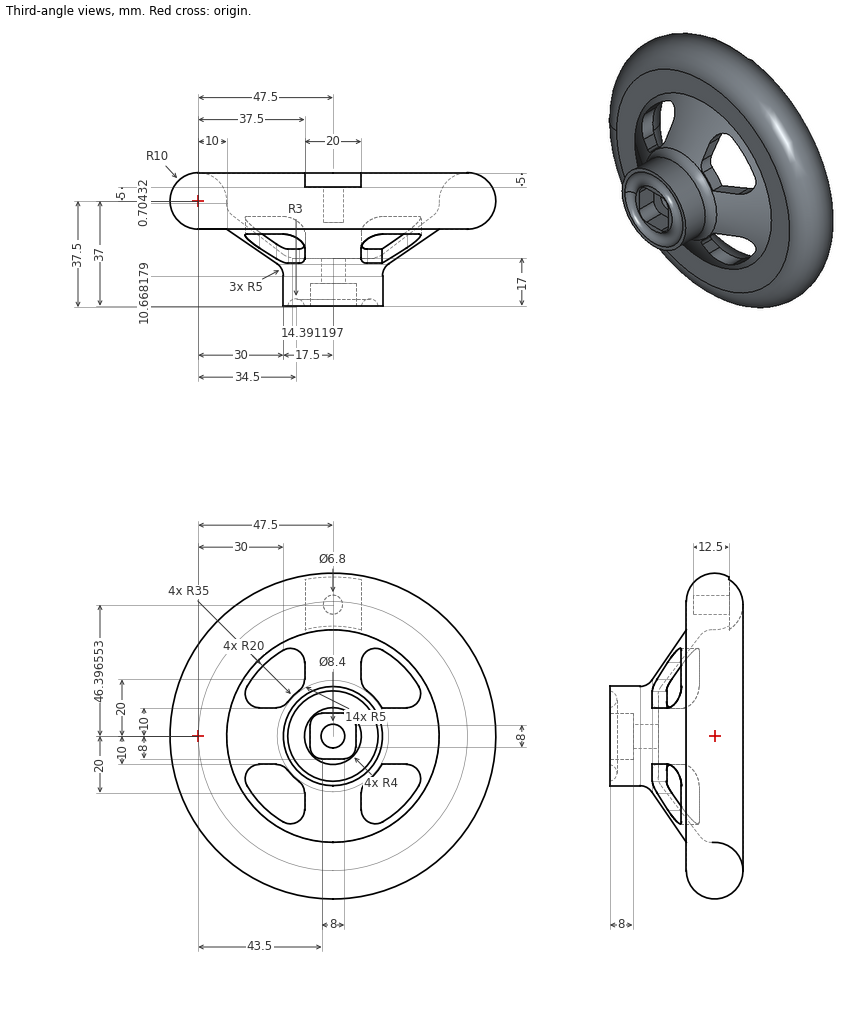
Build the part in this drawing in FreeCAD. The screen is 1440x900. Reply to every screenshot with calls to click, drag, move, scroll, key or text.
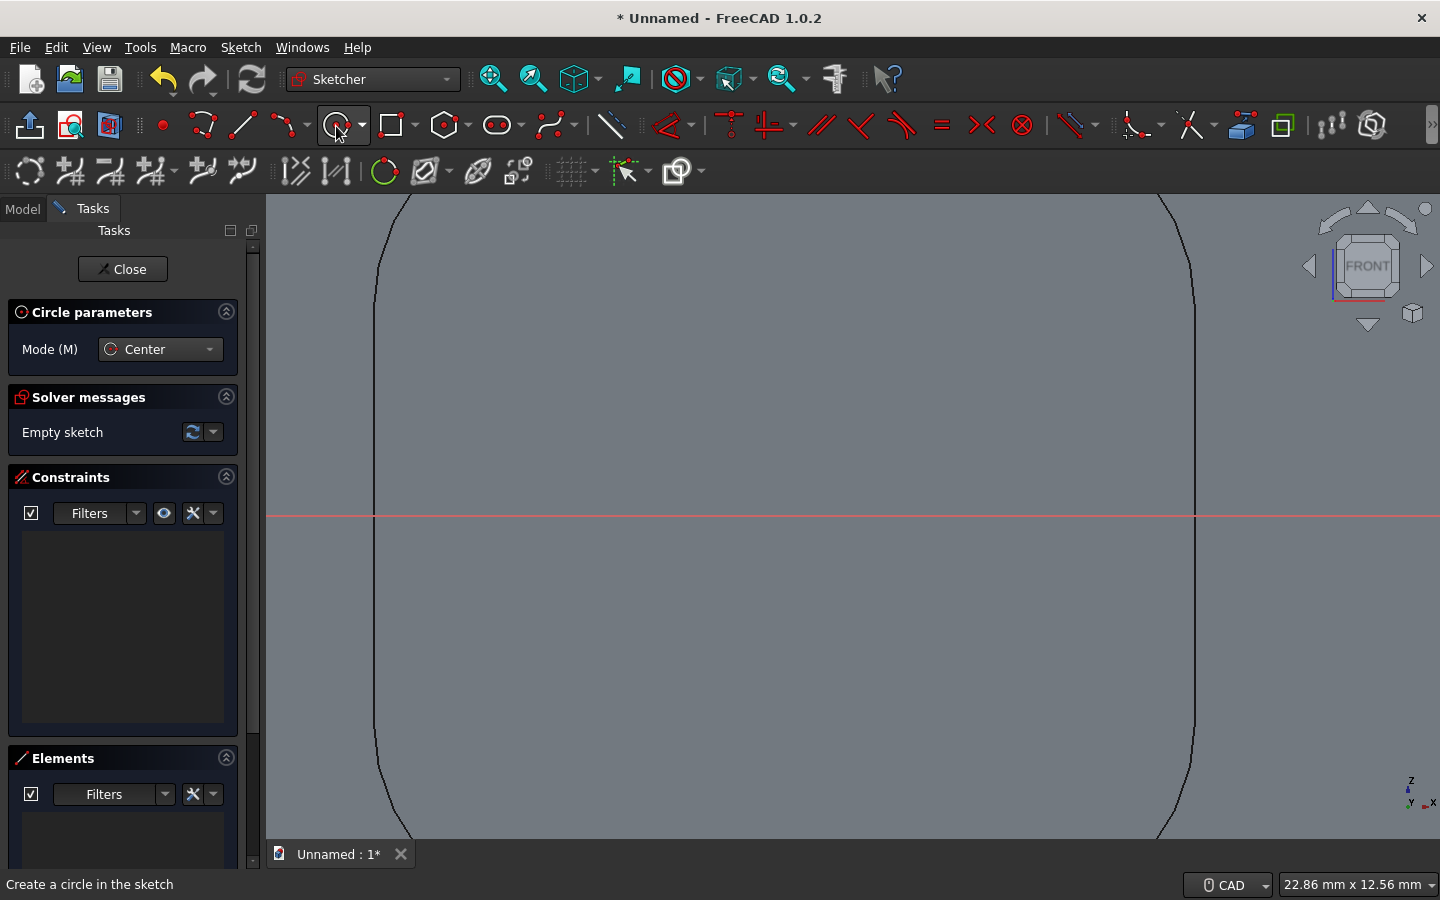
click(784, 516)
move(937, 363)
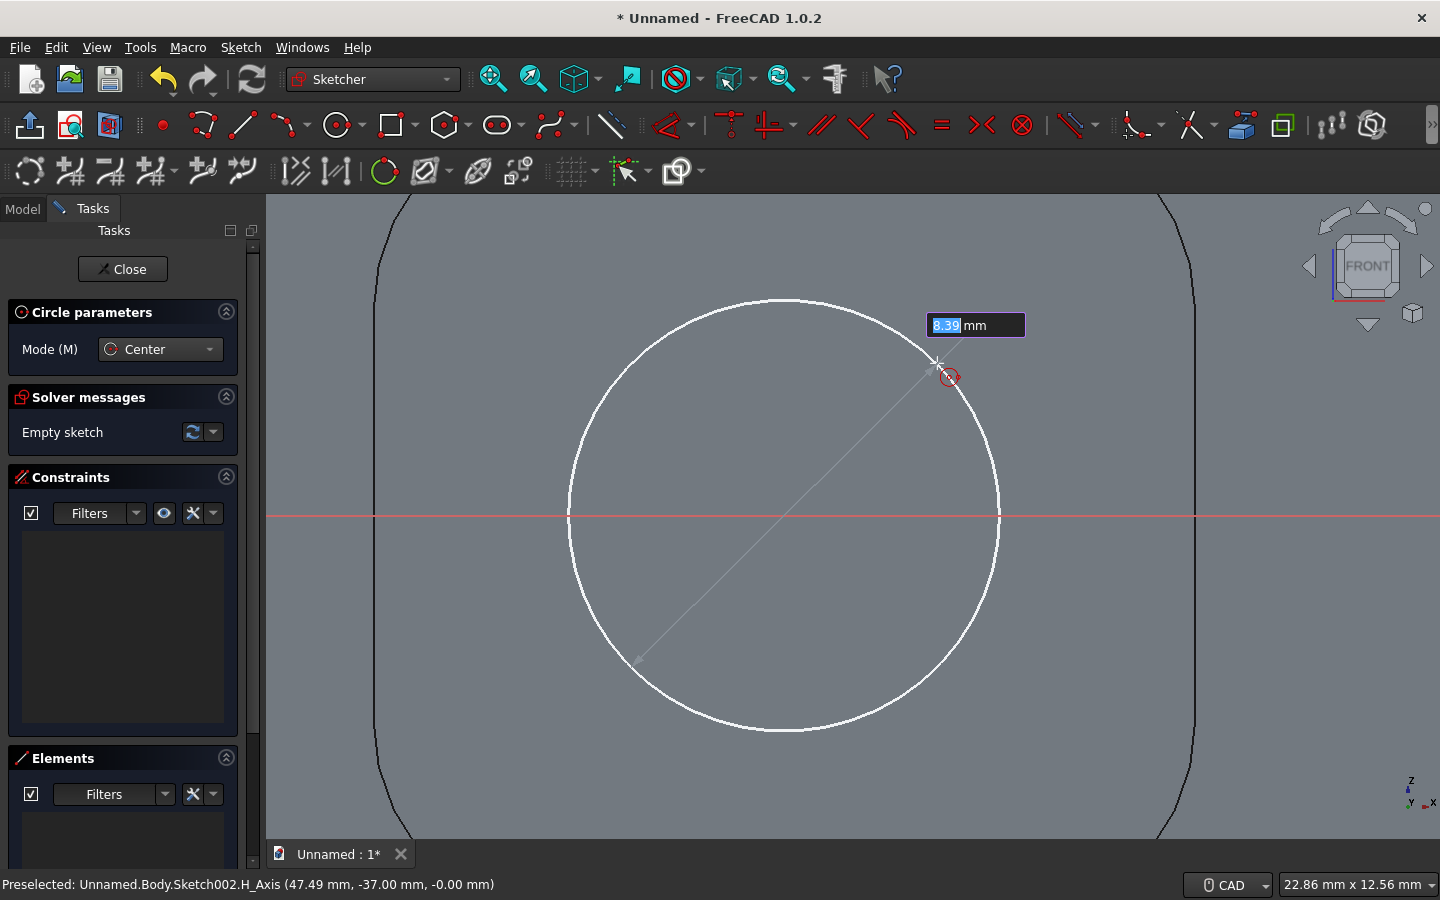
text(8.4)
key(Return)
key(Escape)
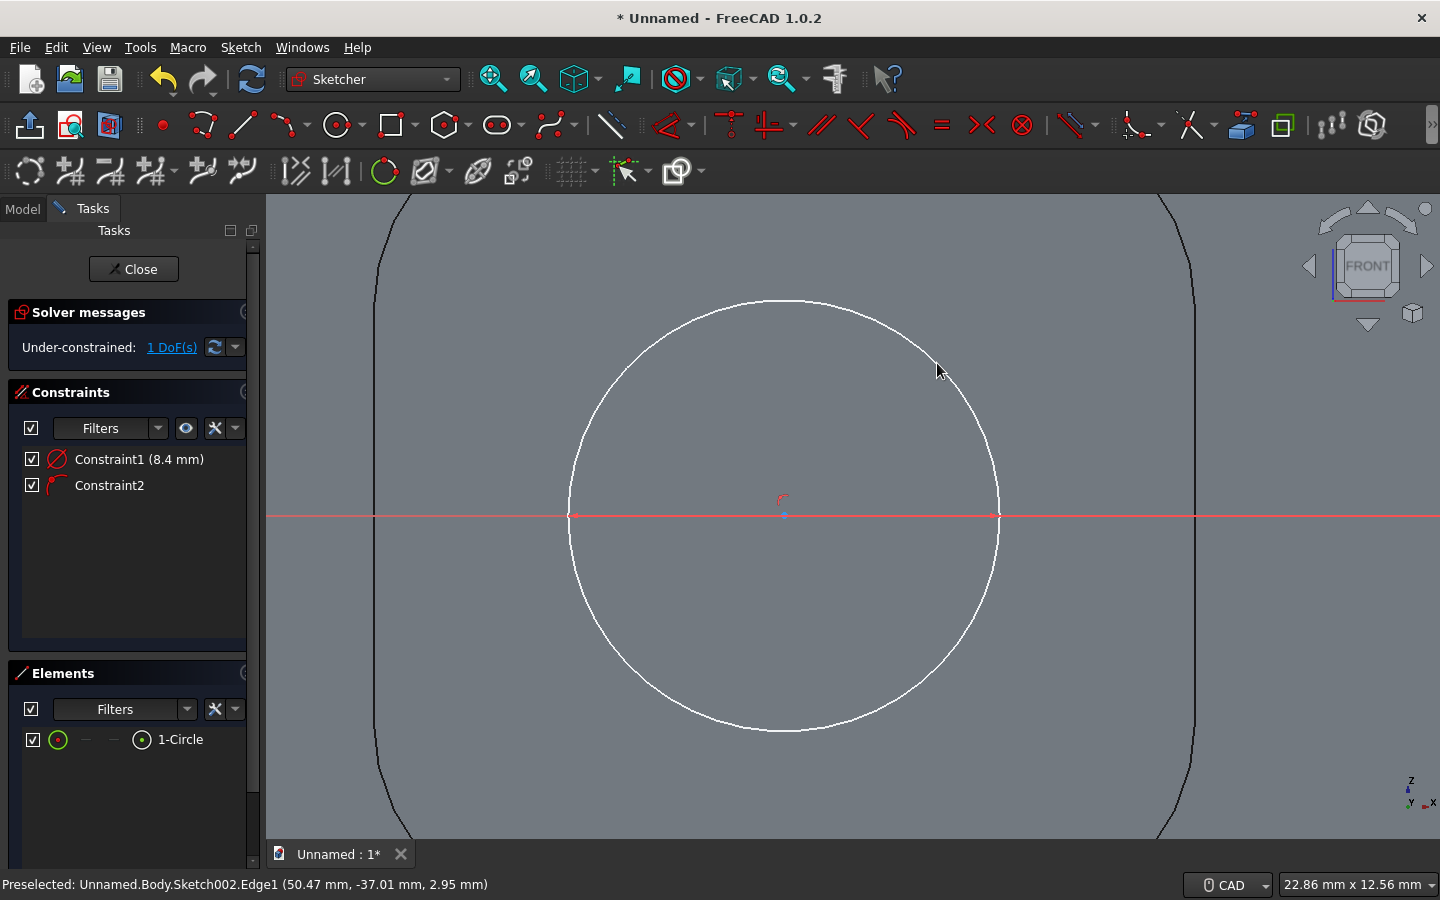
click(666, 126)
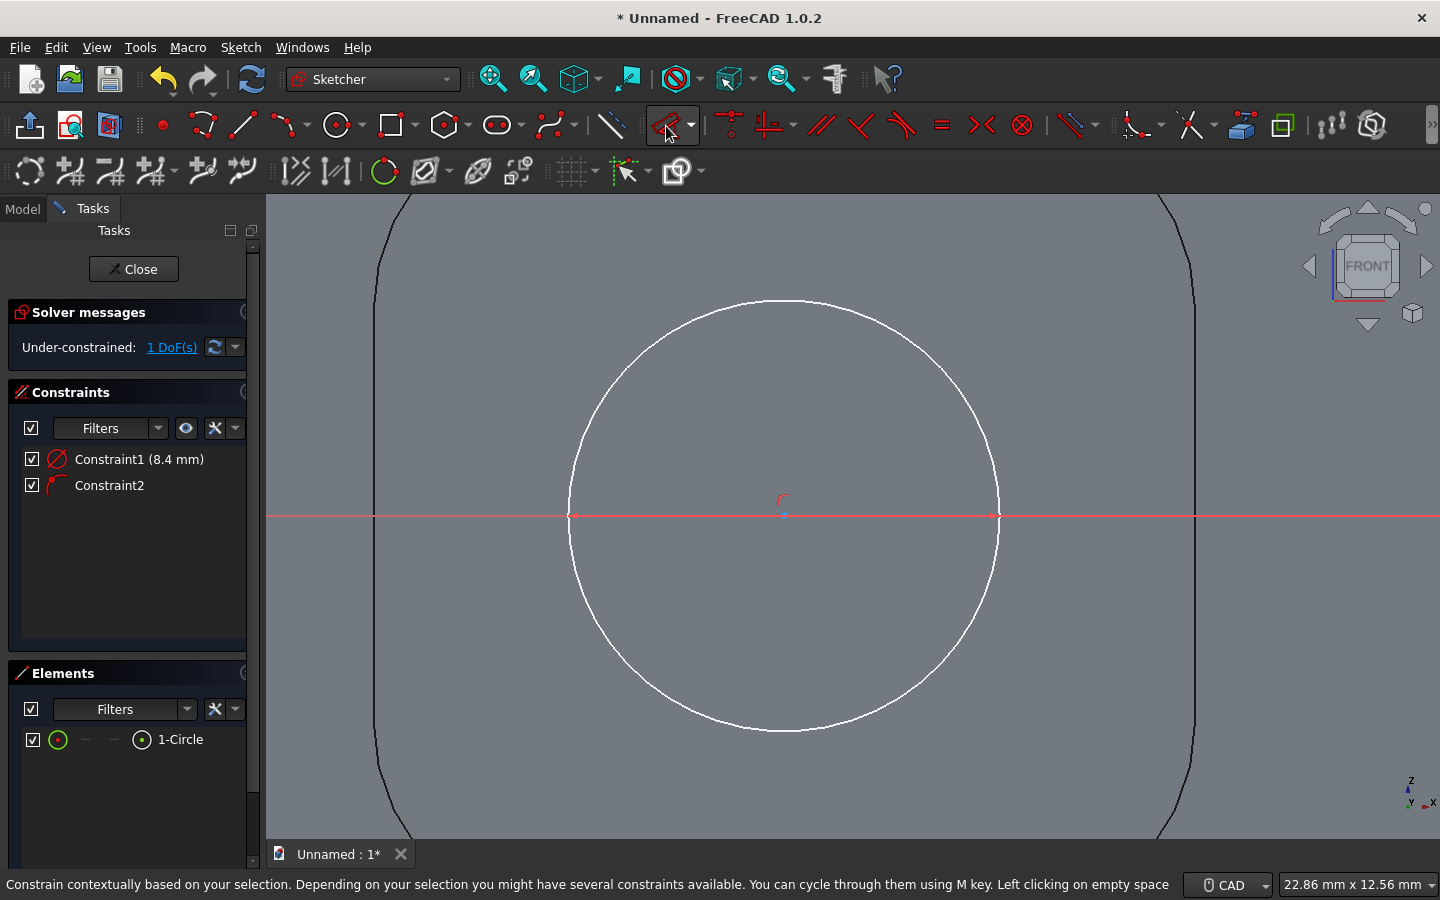
click(784, 516)
click(539, 550)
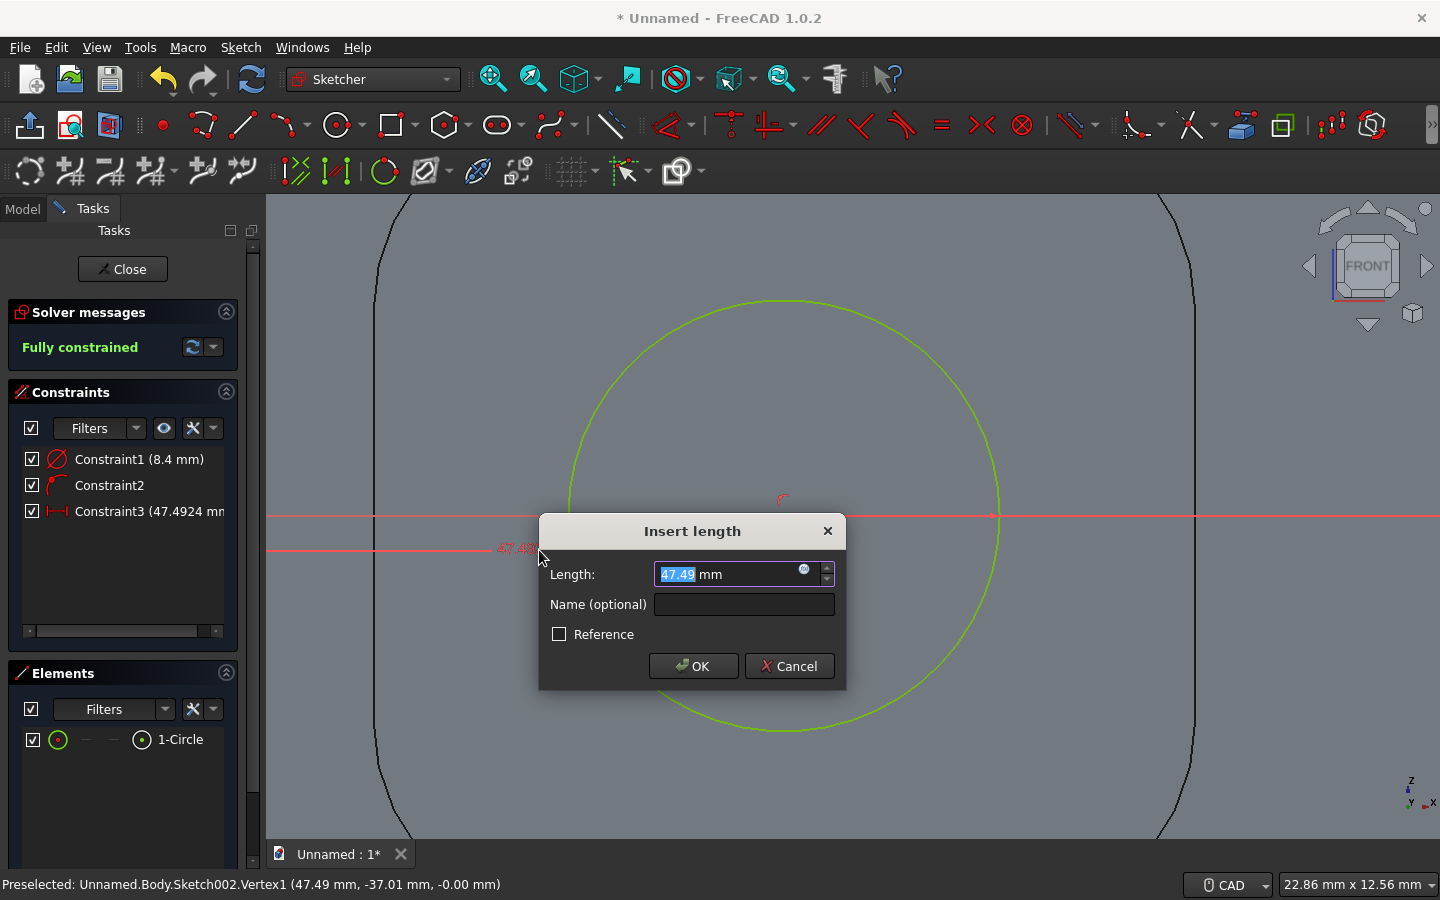
text(47.5)
key(Return)
key(Escape)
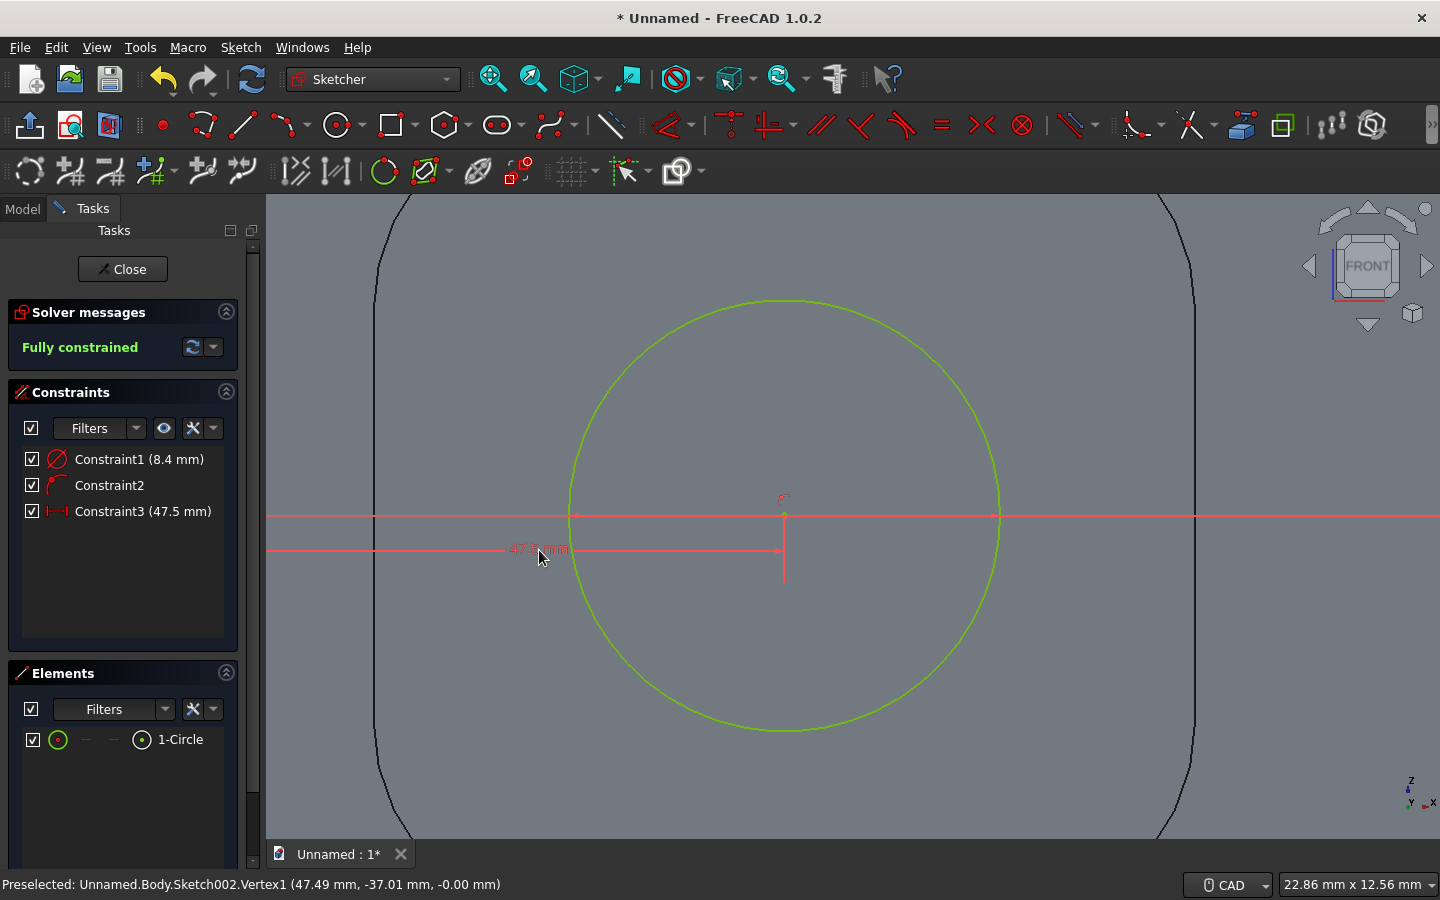
click(123, 269)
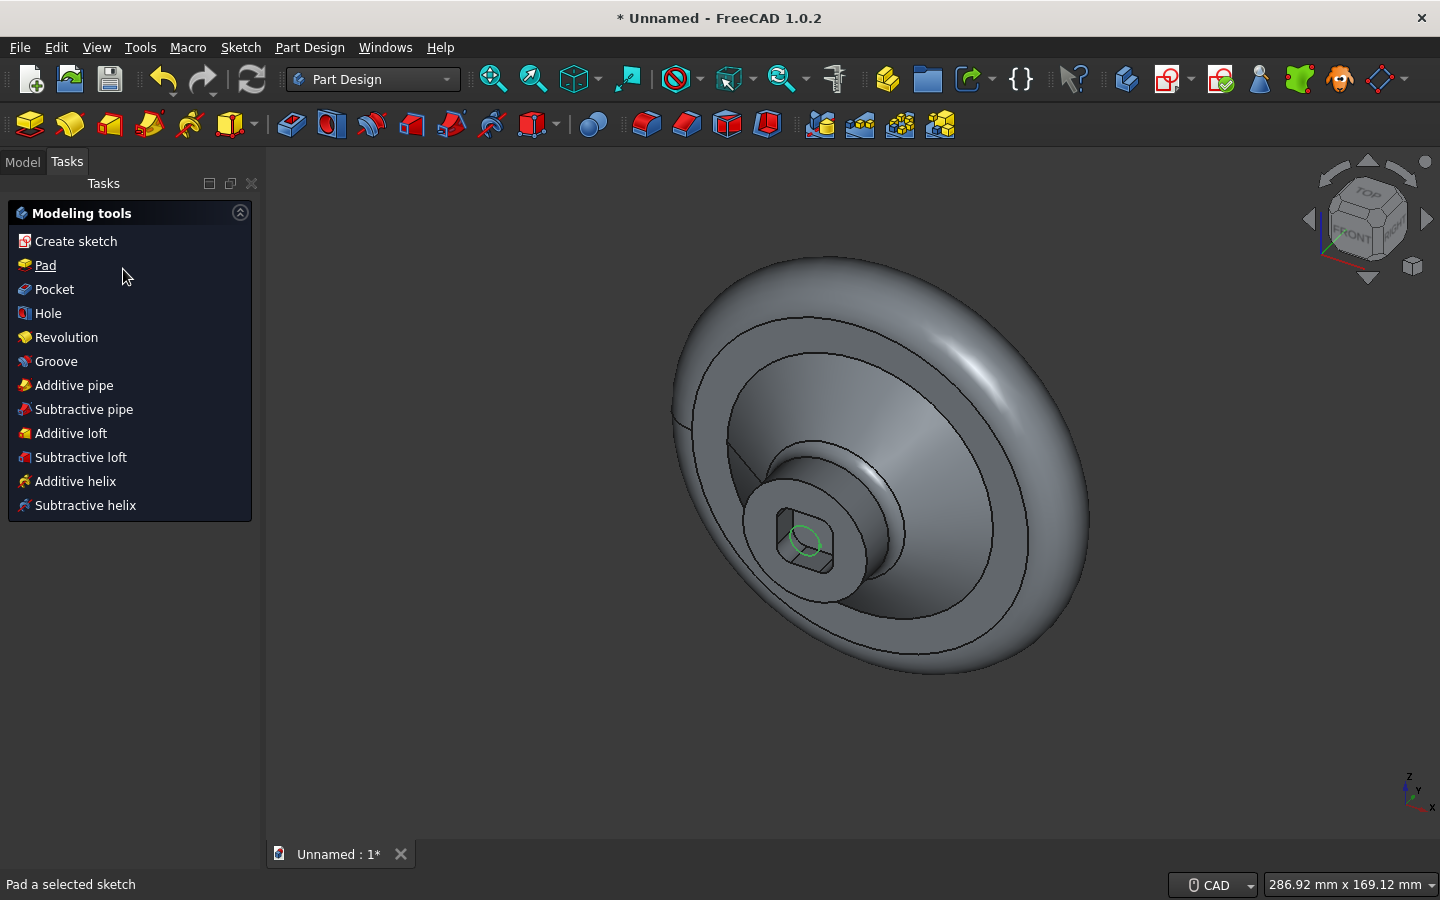
click(292, 124)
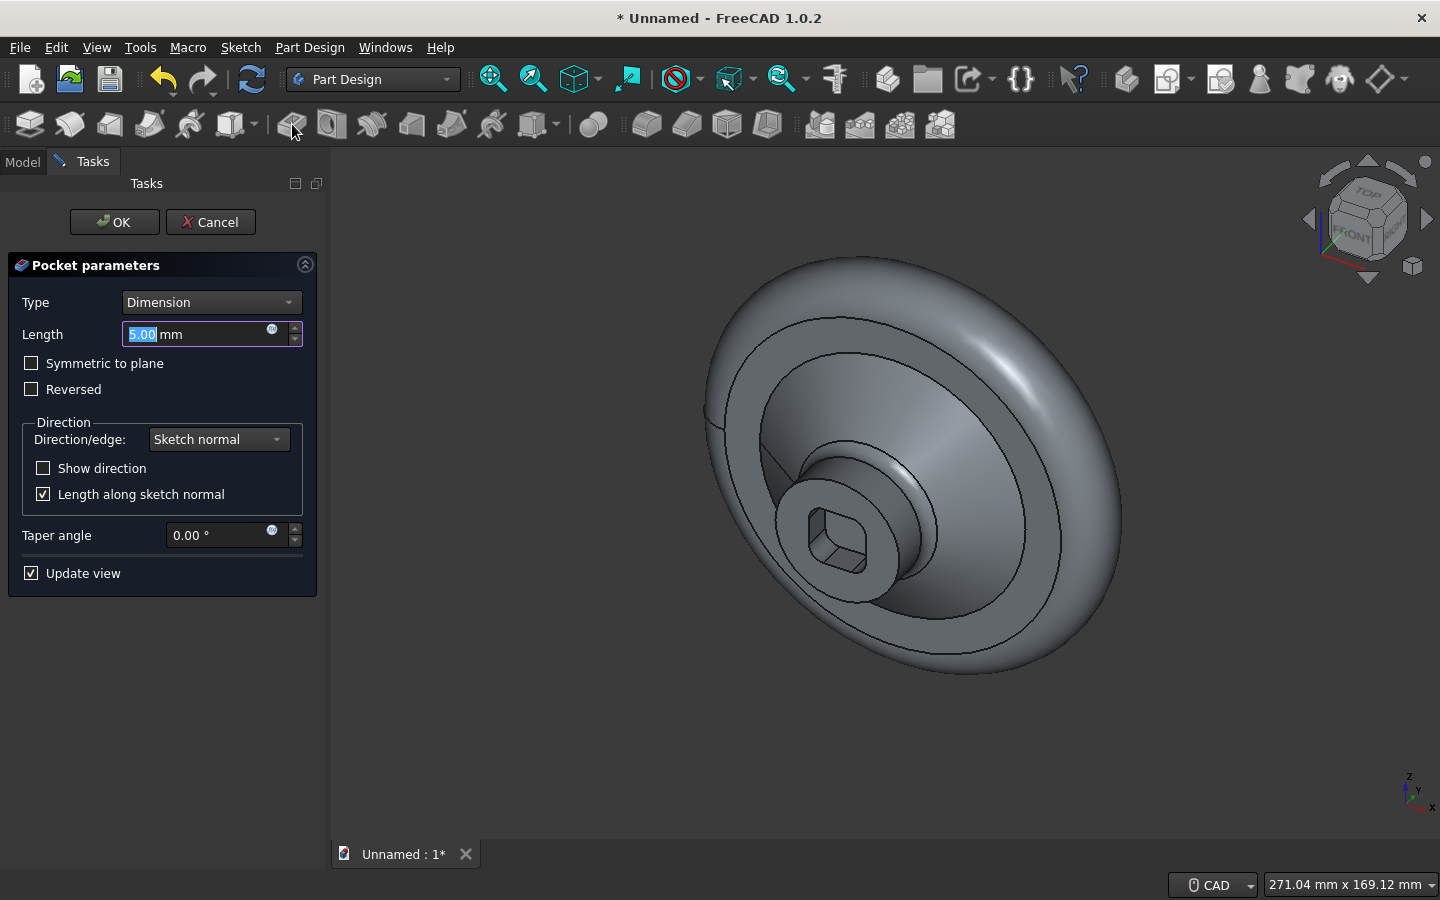
click(212, 302)